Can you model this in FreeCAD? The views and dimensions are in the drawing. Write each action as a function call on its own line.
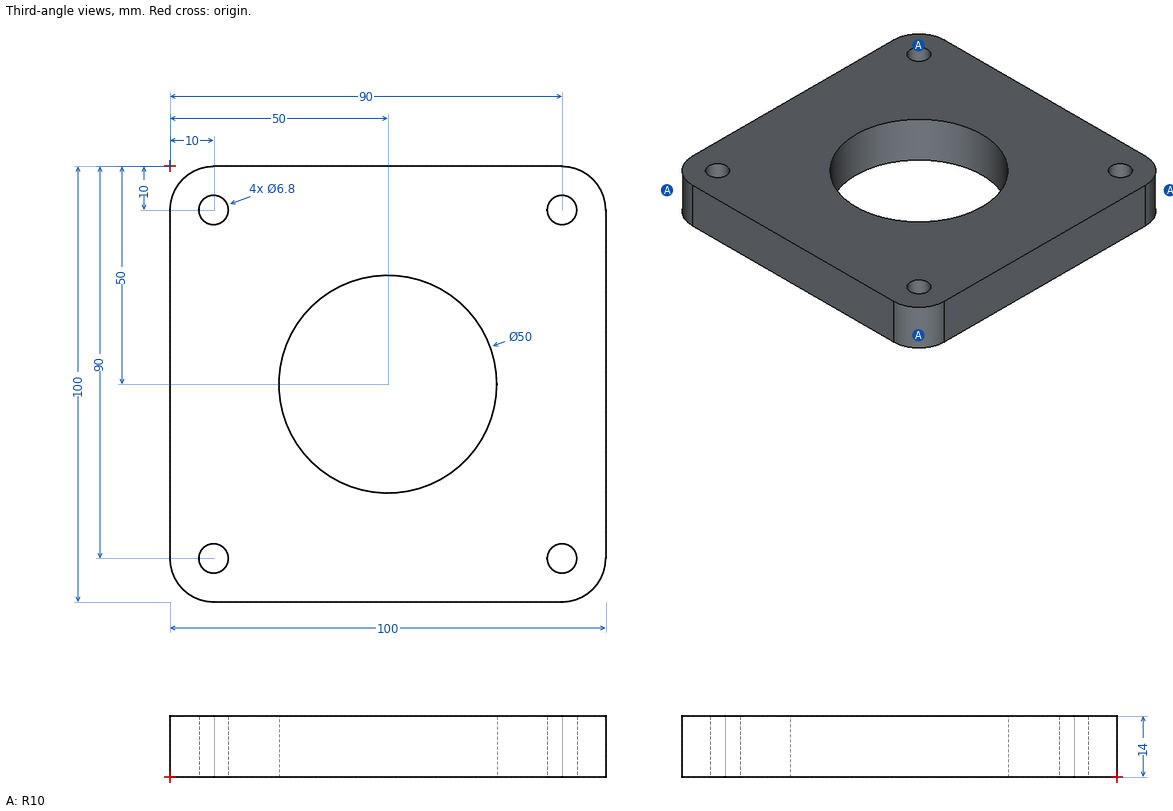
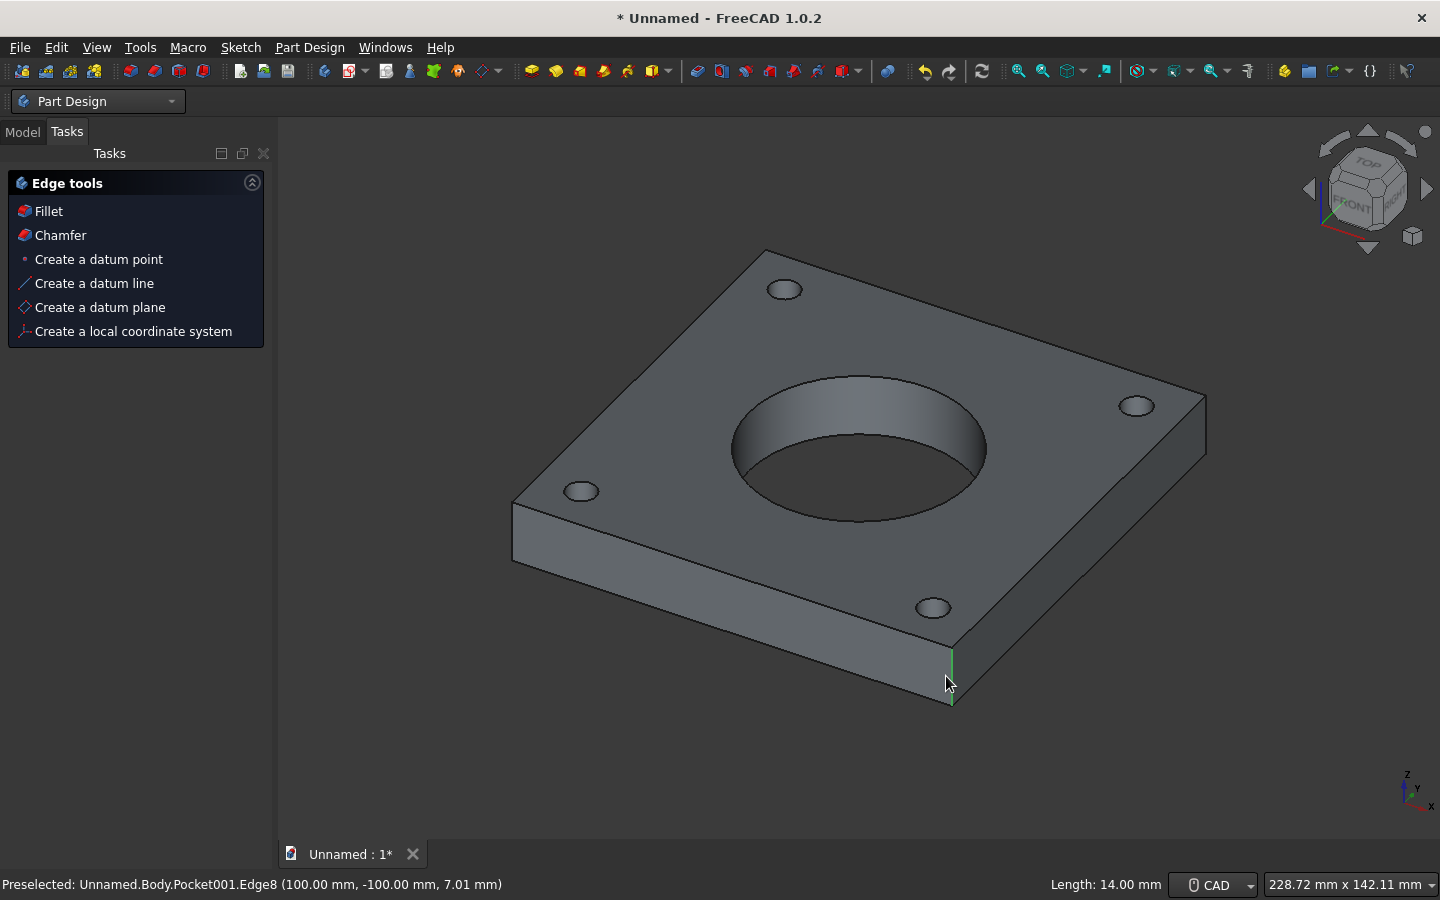
key(0)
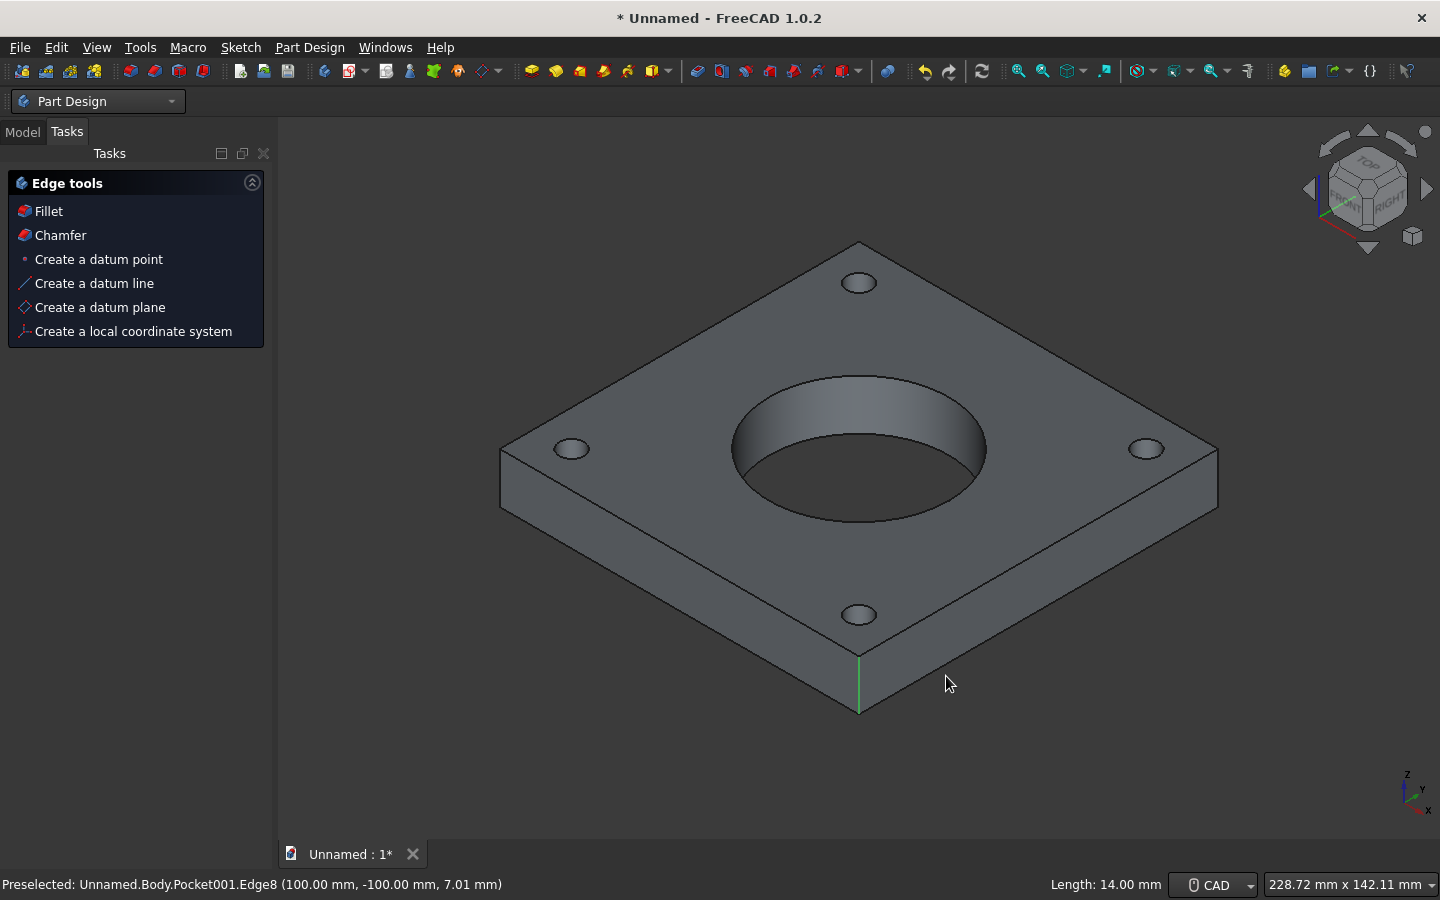
key(2)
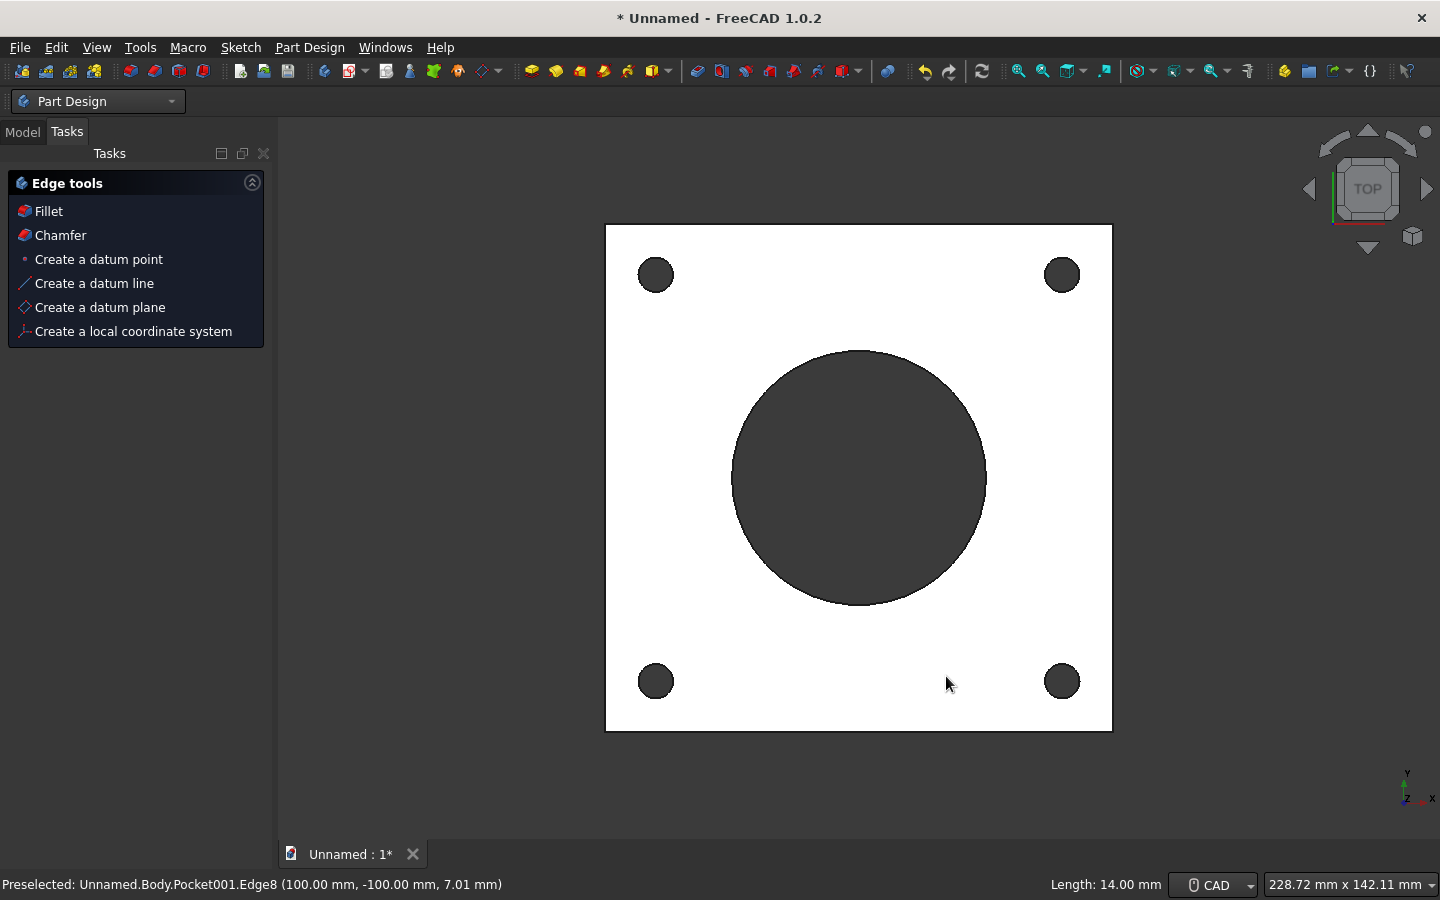
key(1)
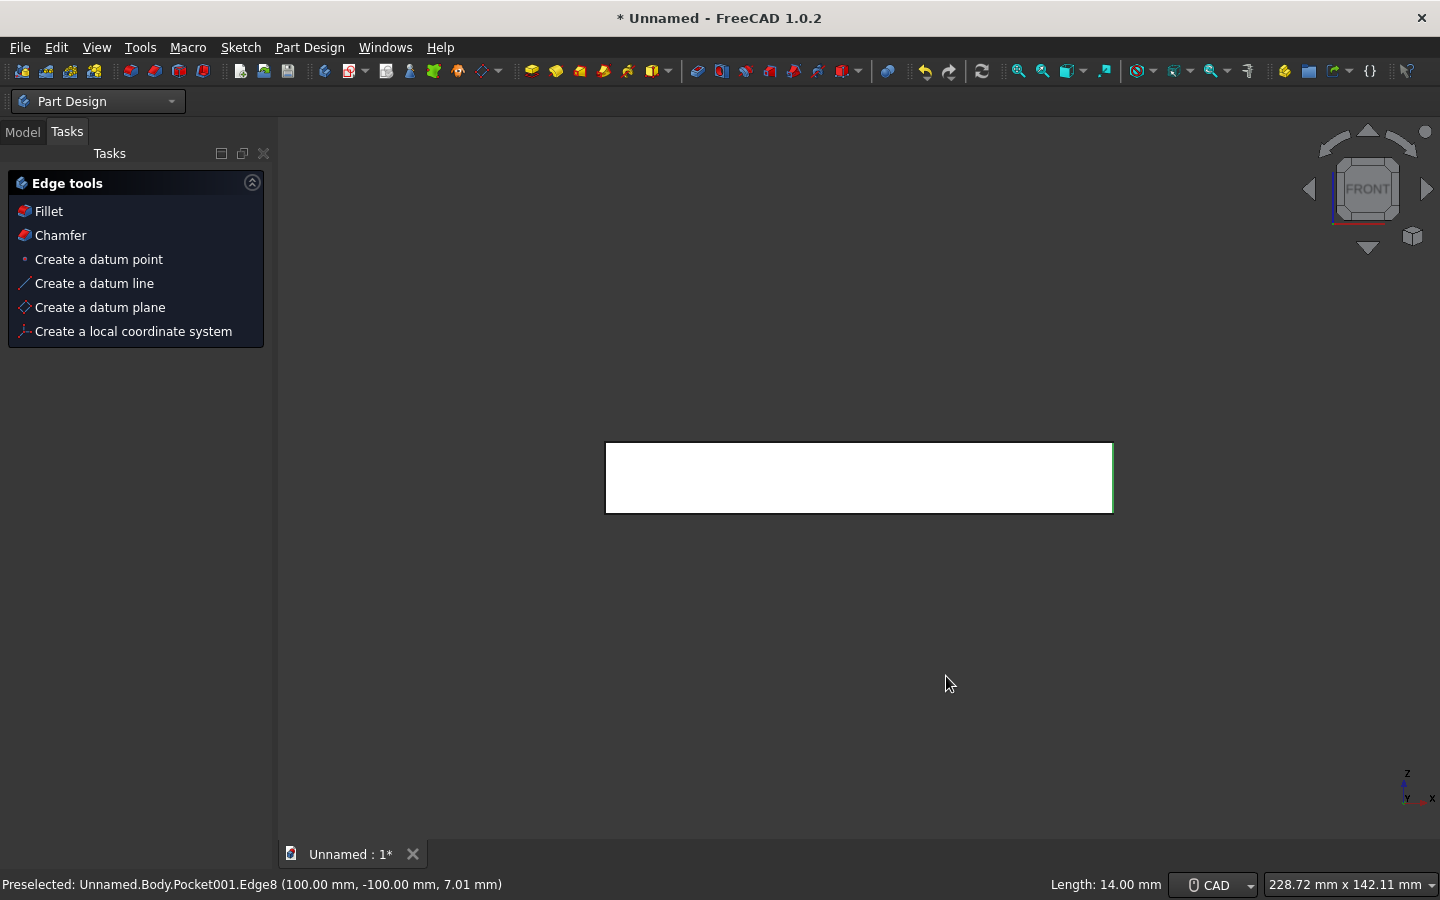
click(1020, 72)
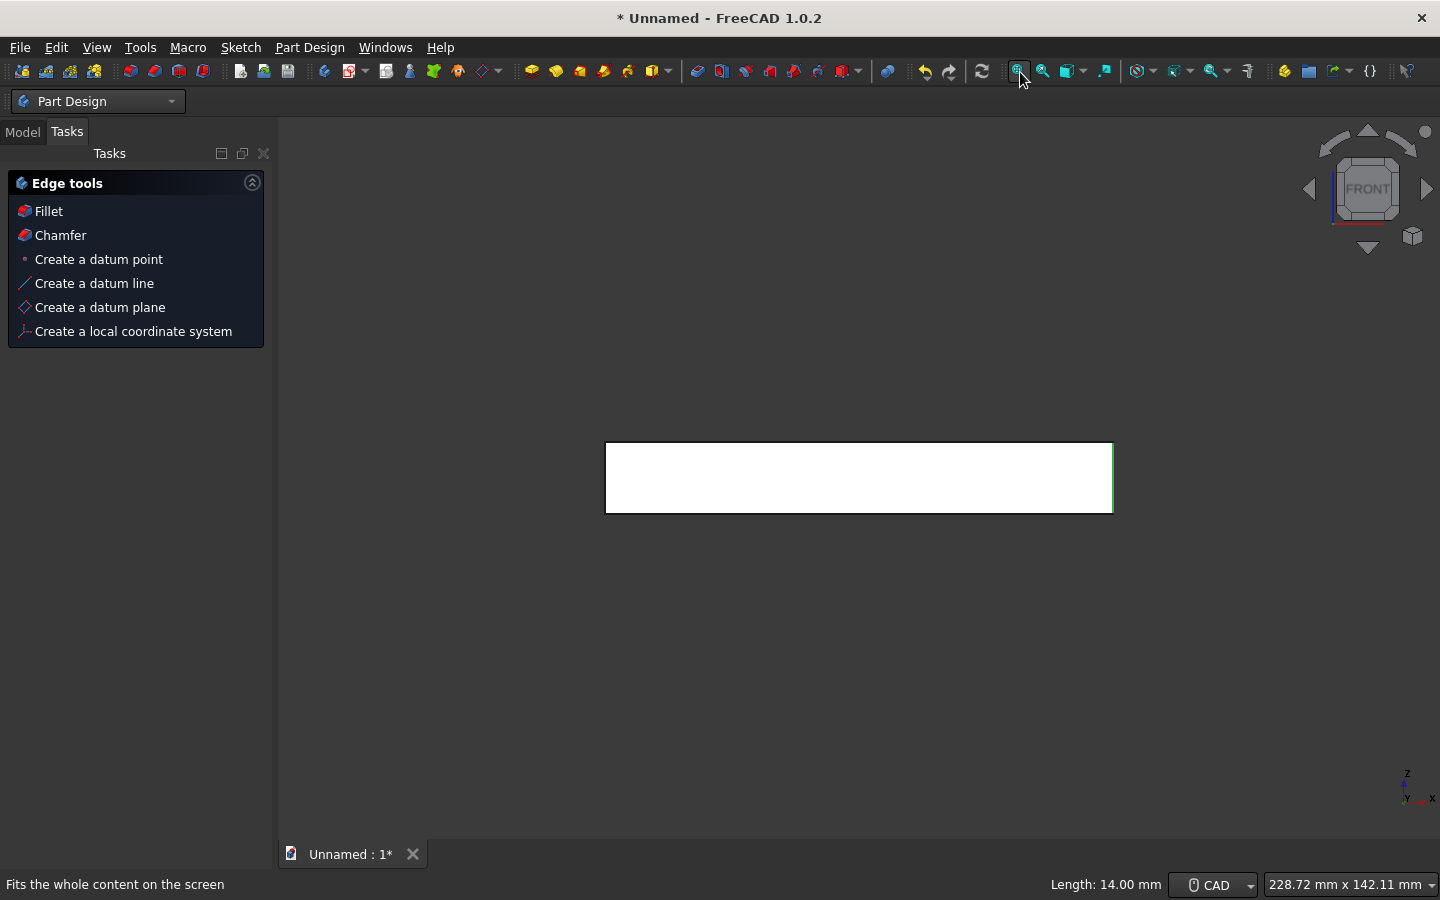
click(605, 477, ctrl)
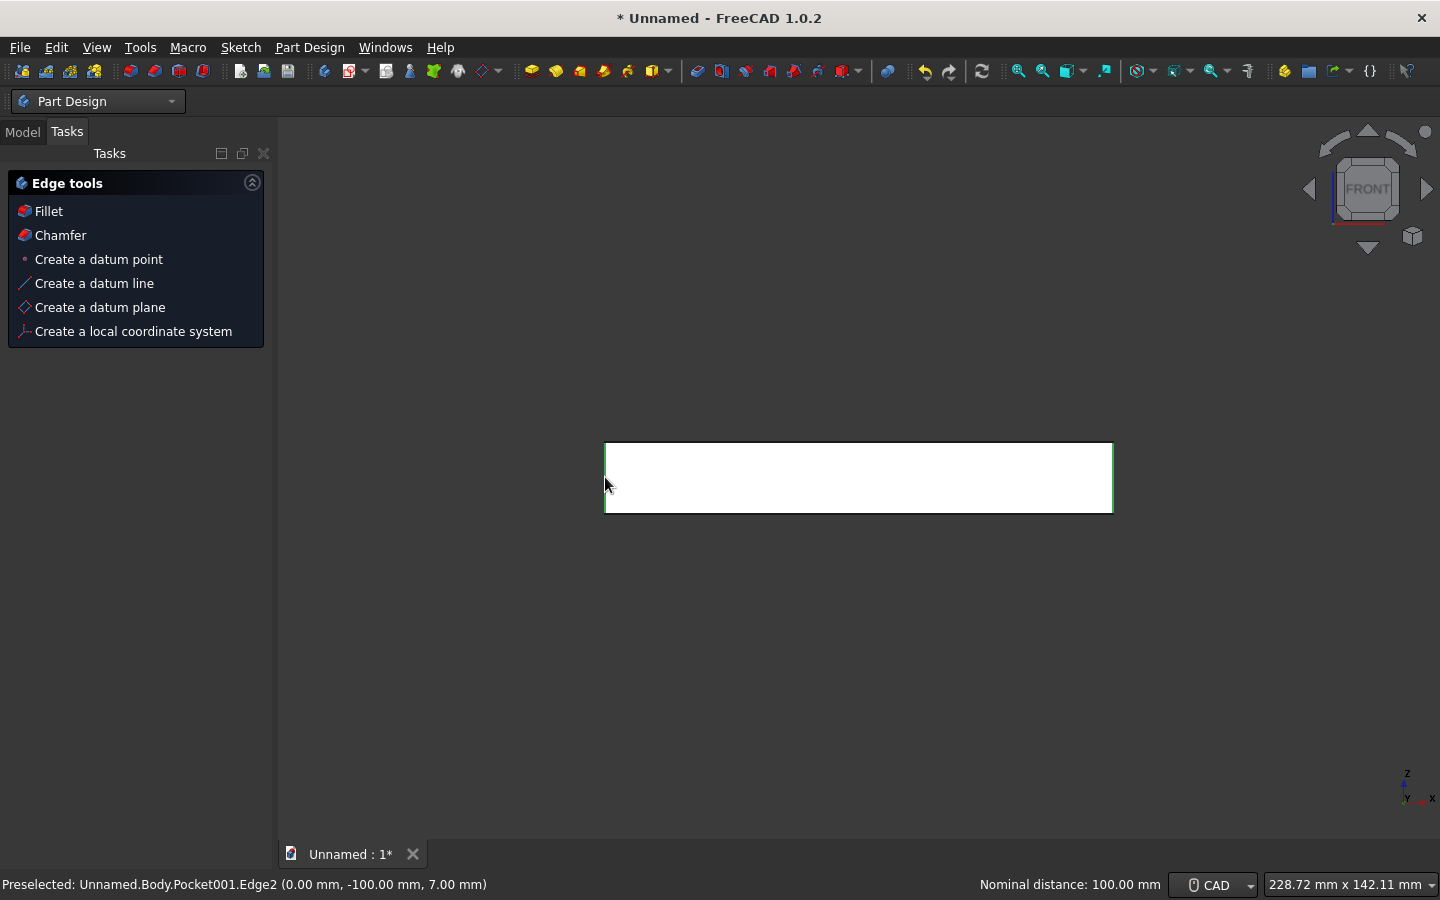
key(3)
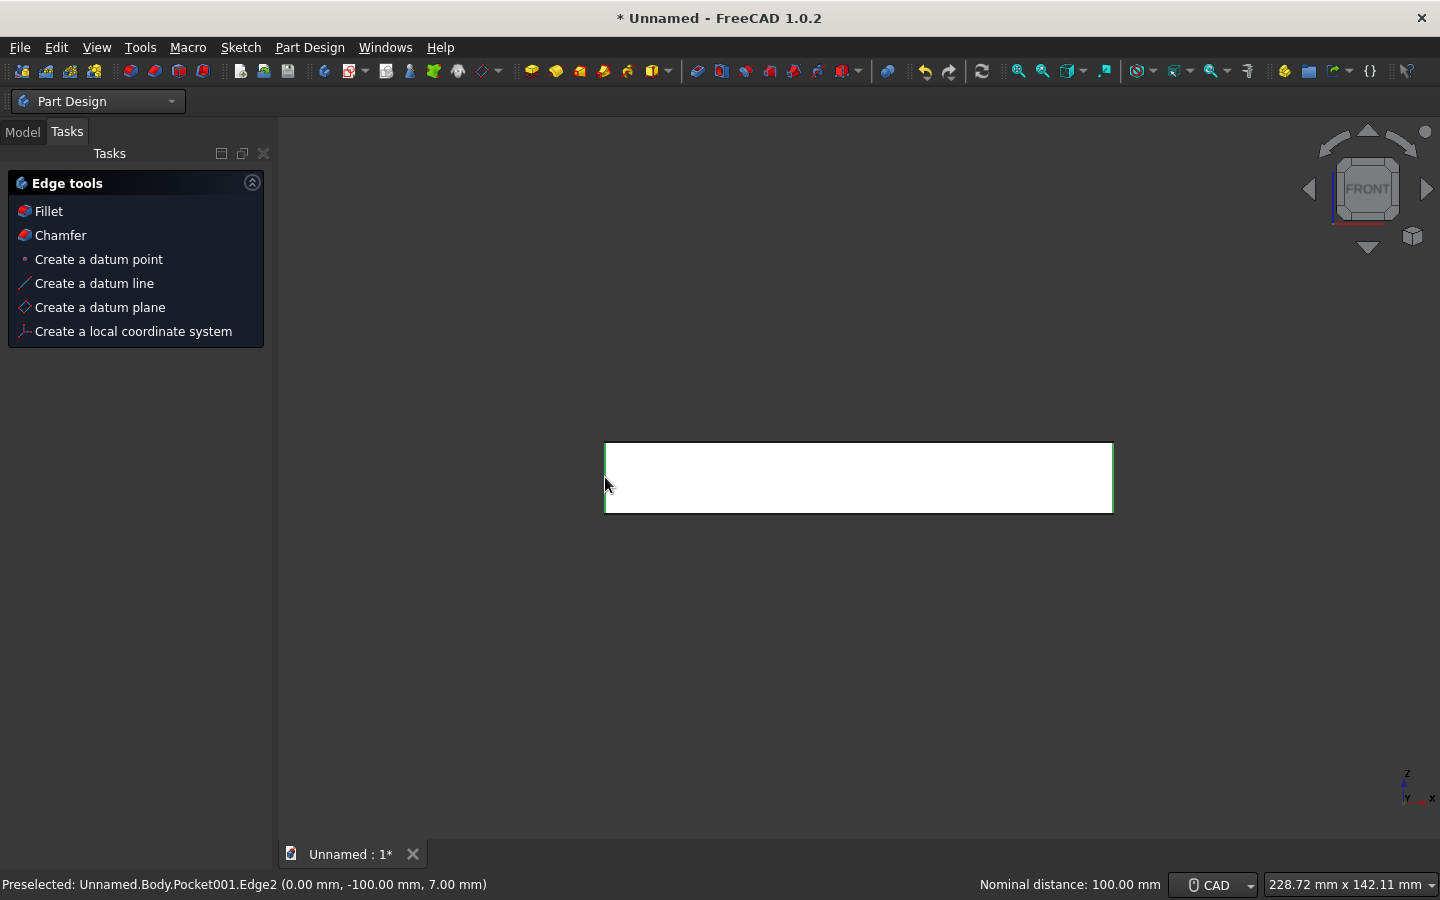
click(1020, 72)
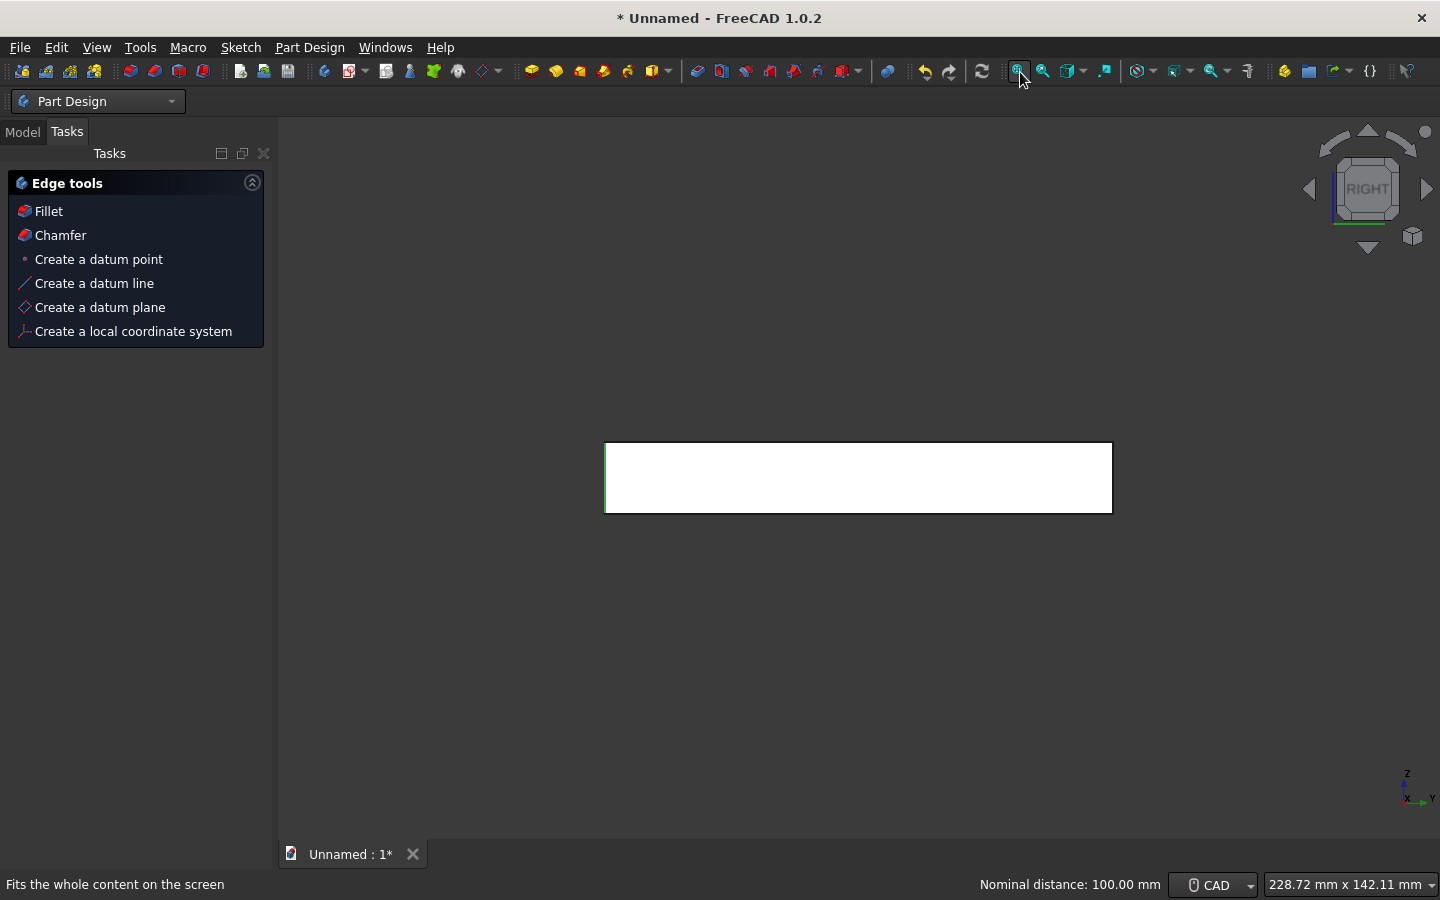
click(1113, 477, ctrl)